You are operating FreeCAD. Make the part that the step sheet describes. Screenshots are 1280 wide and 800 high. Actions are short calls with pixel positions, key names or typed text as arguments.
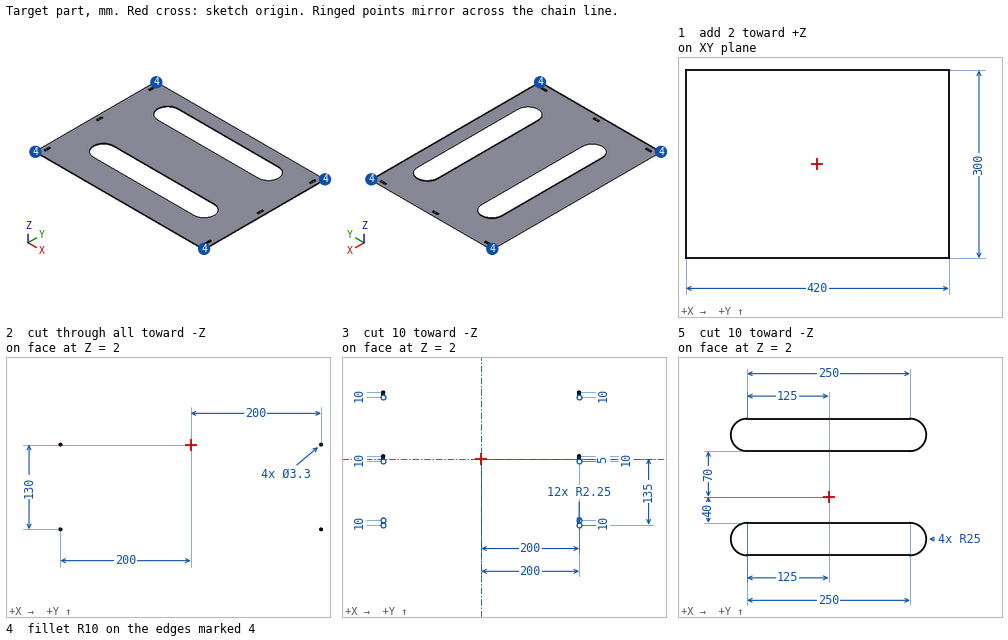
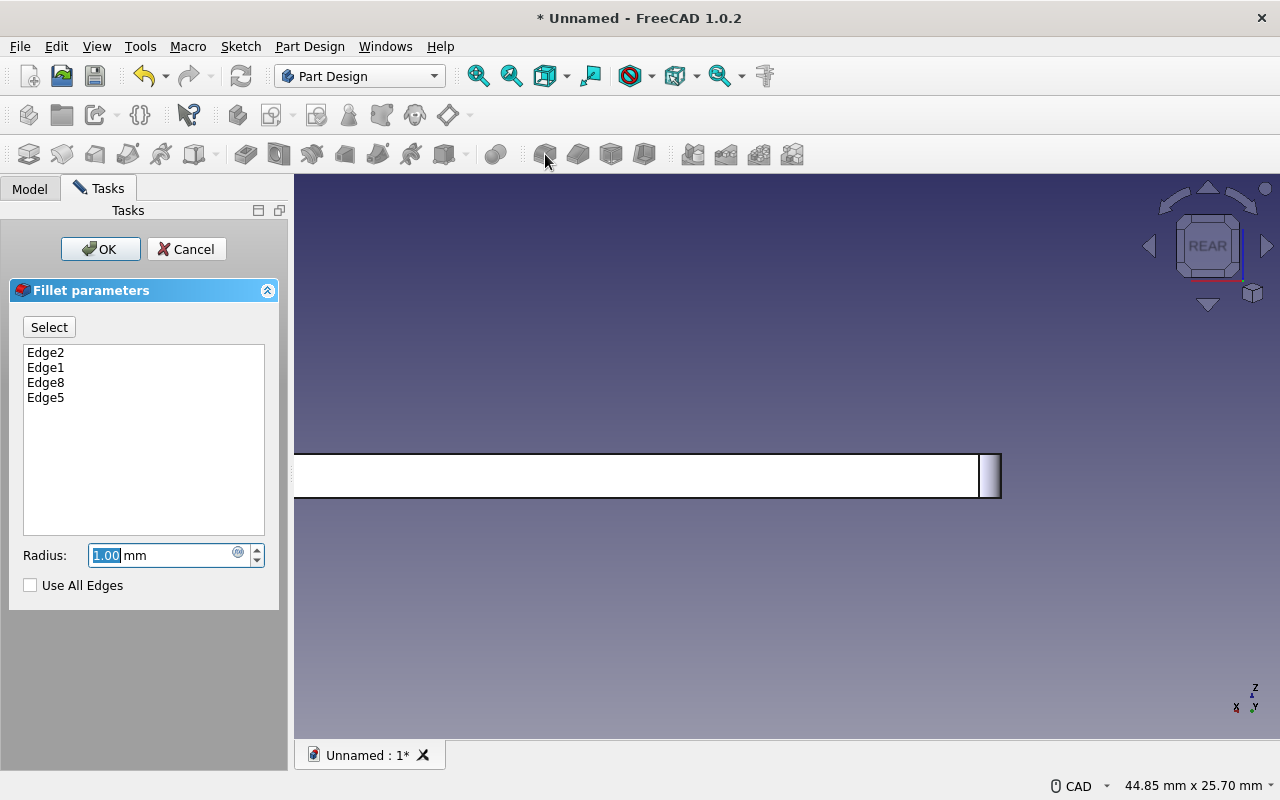
text(10)
key(Tab)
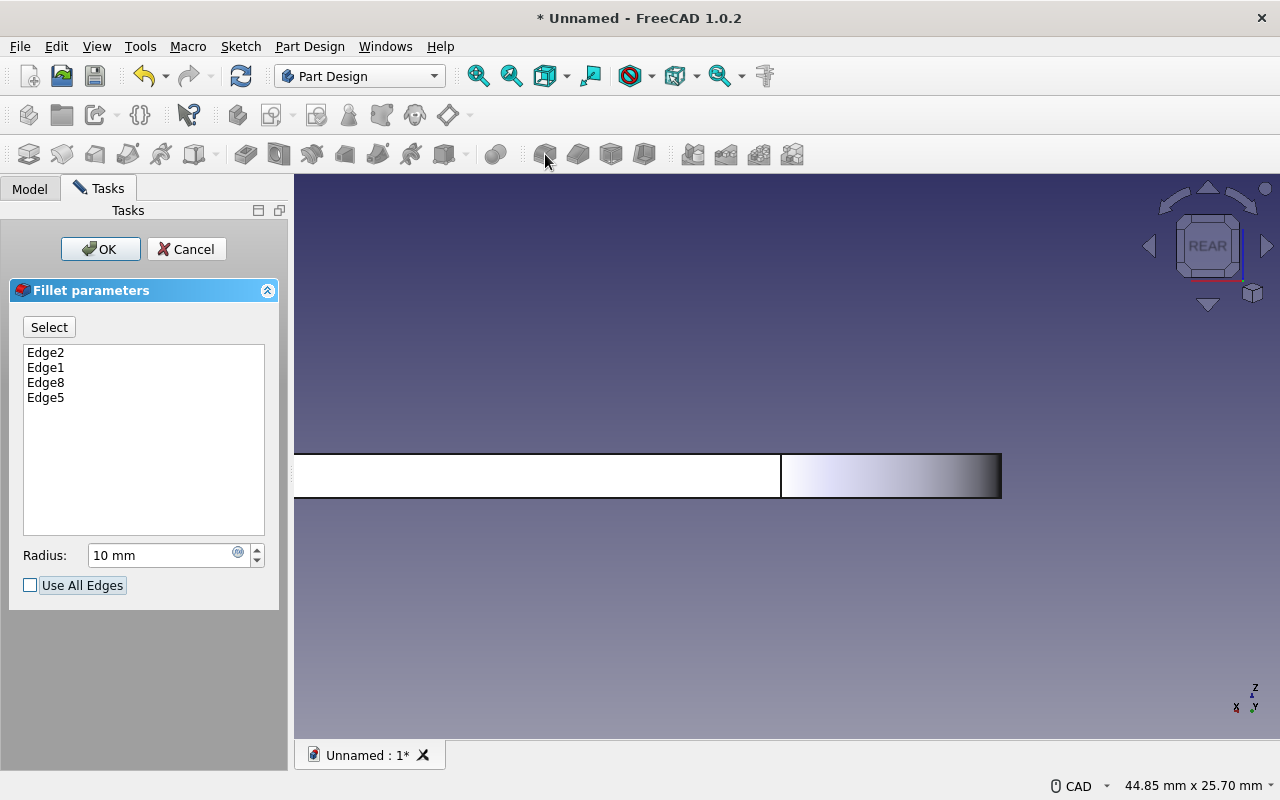
click(101, 249)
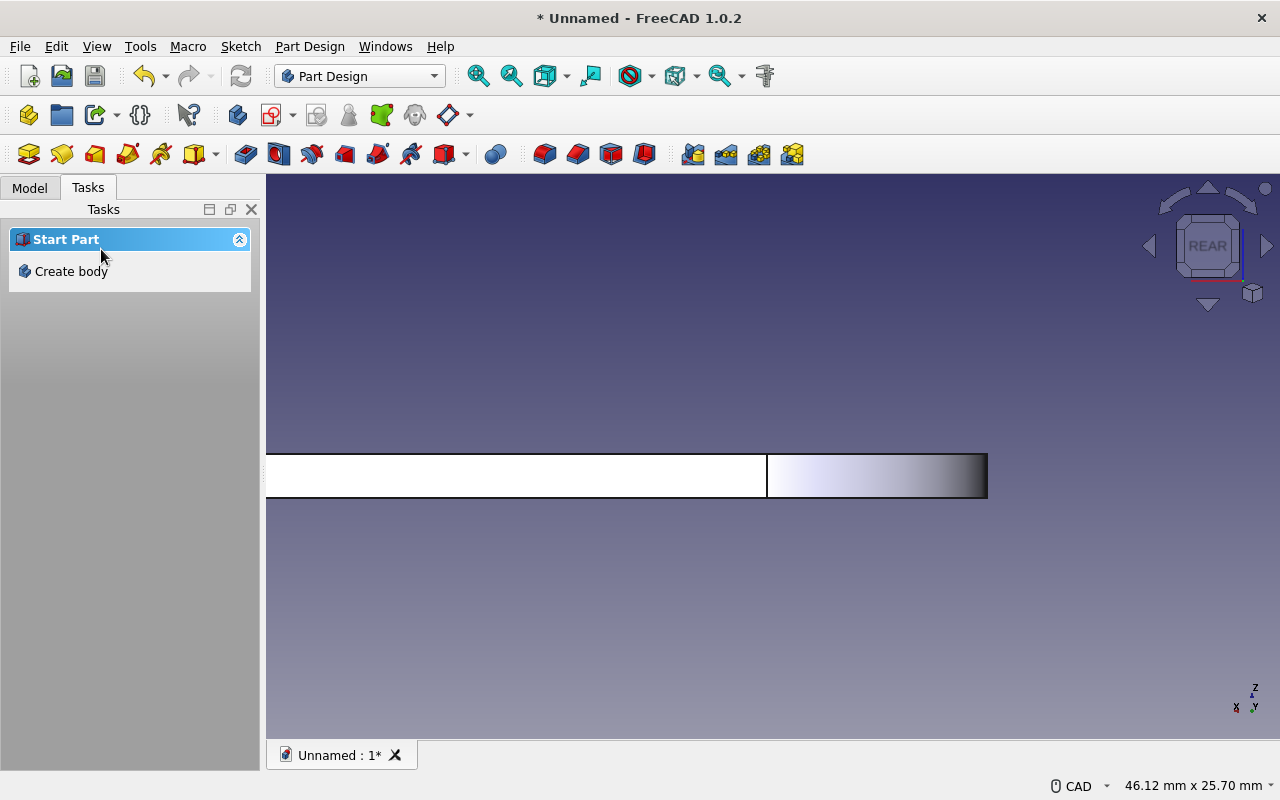
click(479, 76)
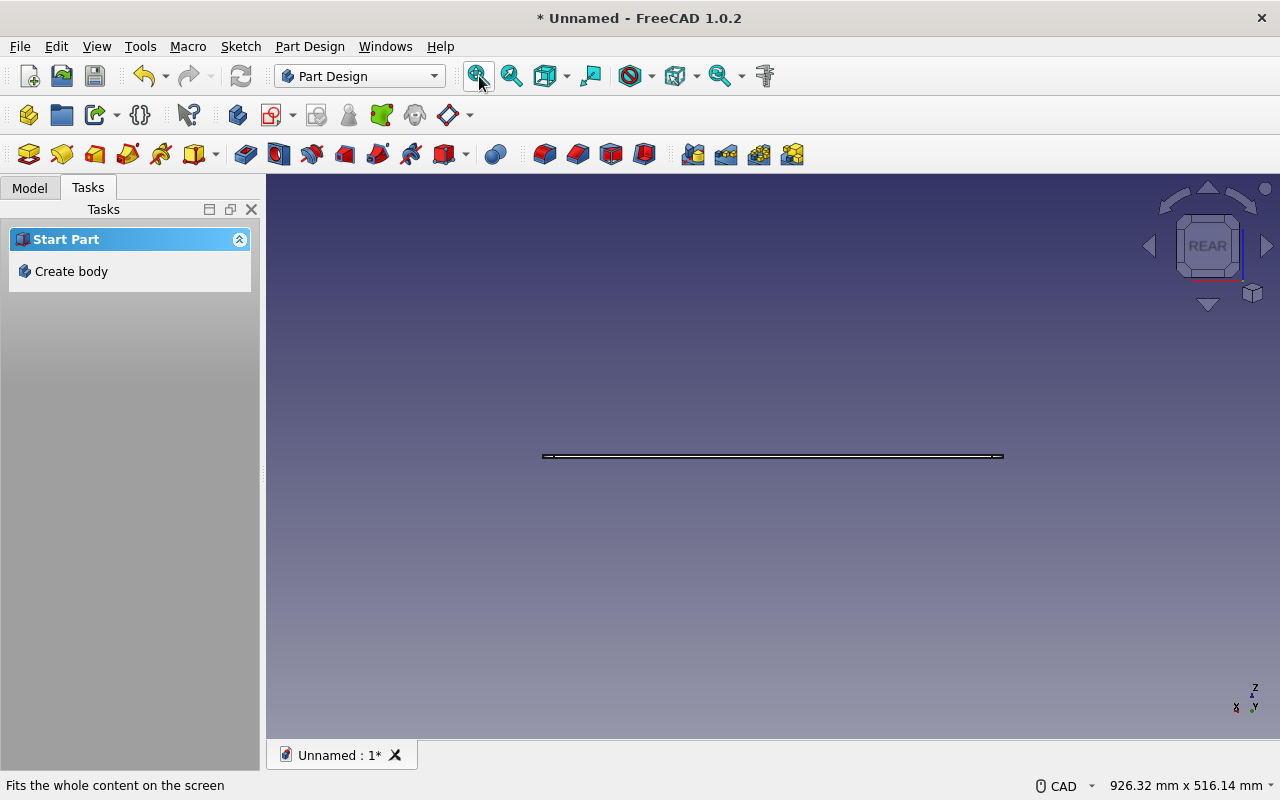
key(0)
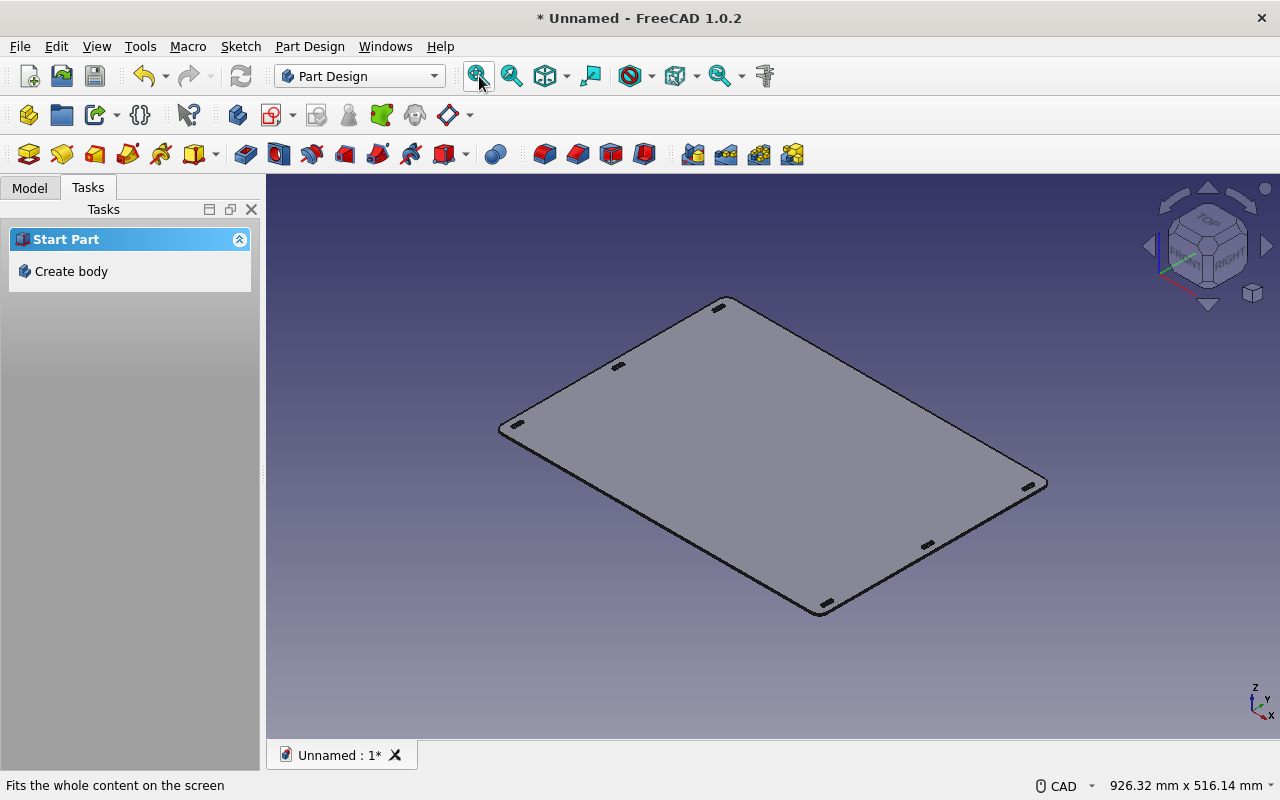
click(773, 455)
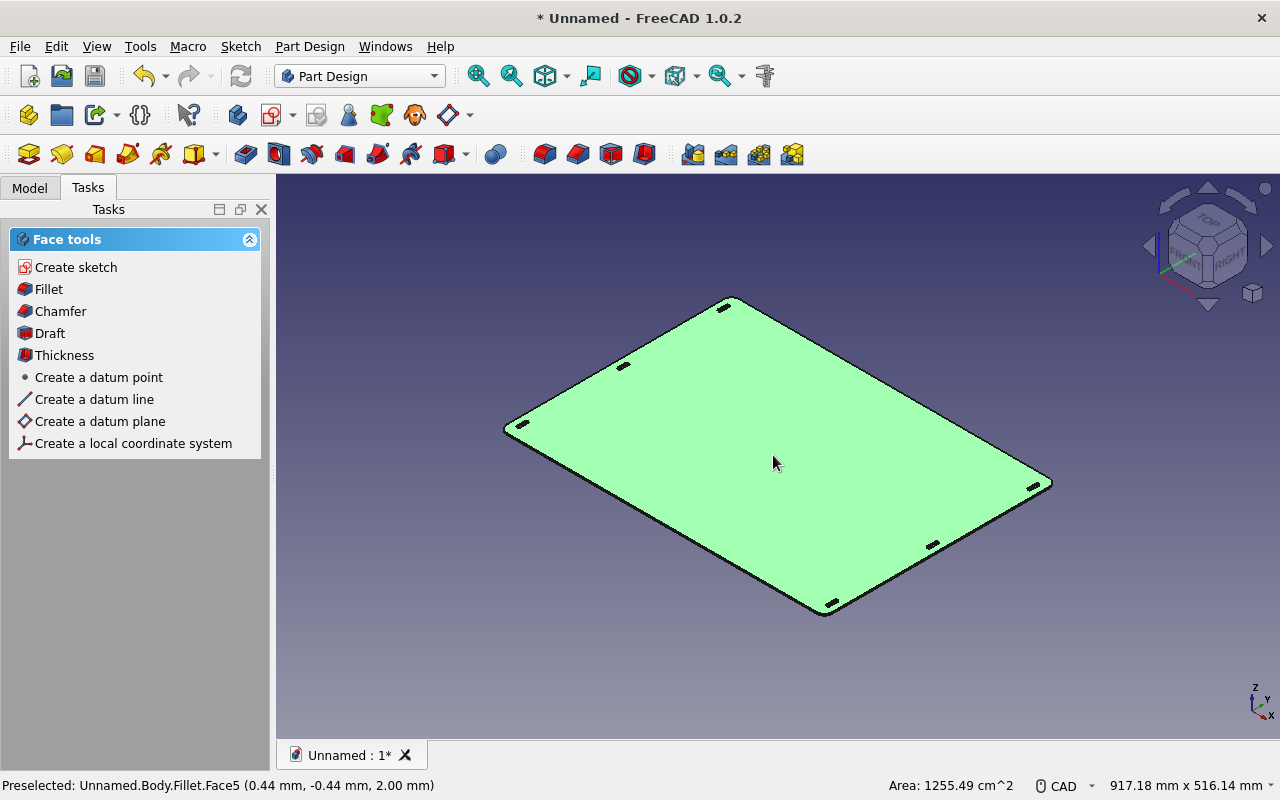
click(270, 116)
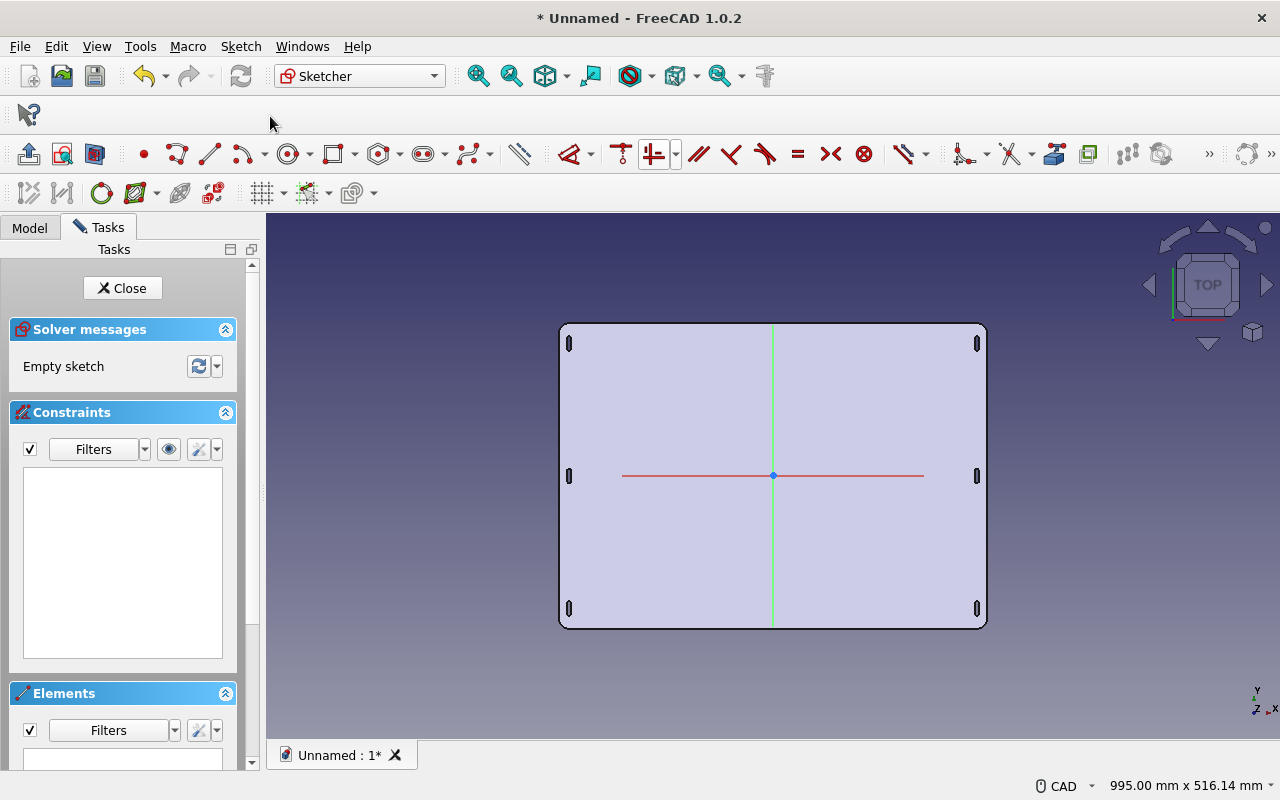
scroll(912, 430, up, 2)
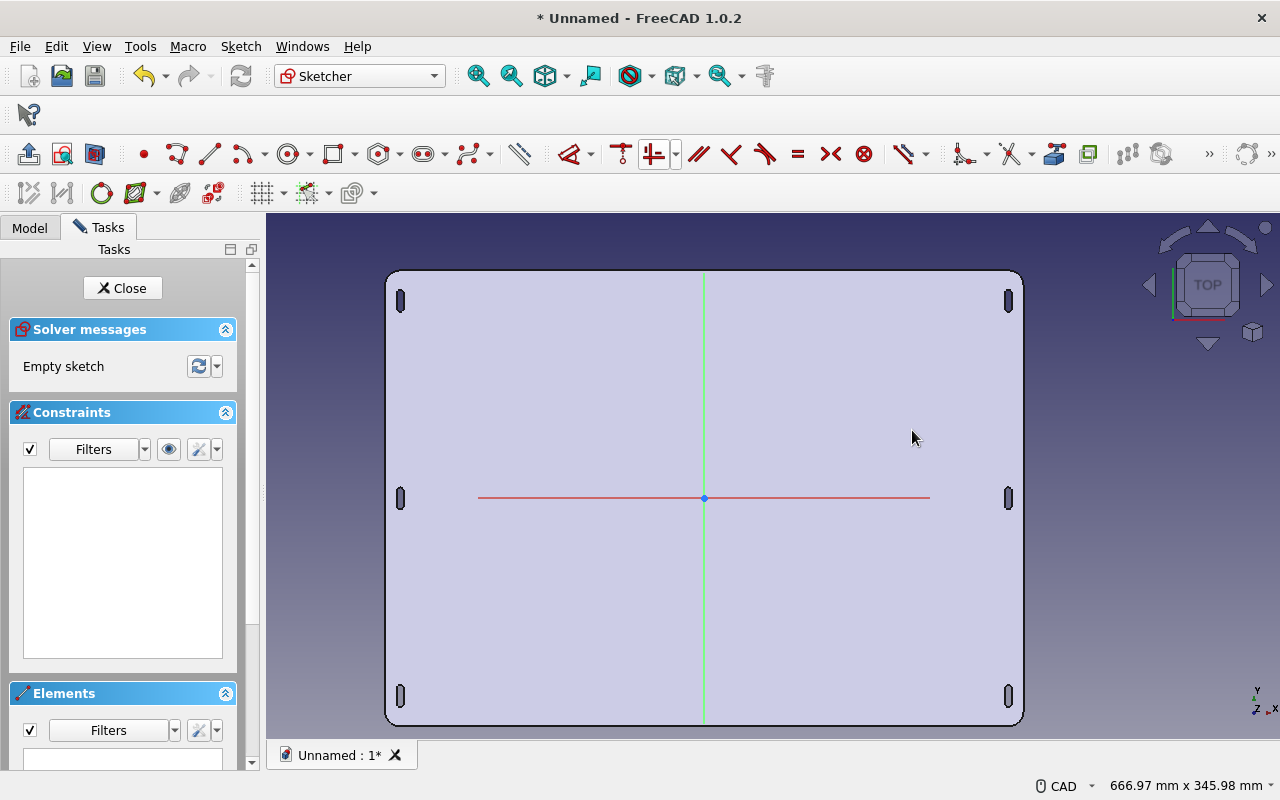
click(422, 154)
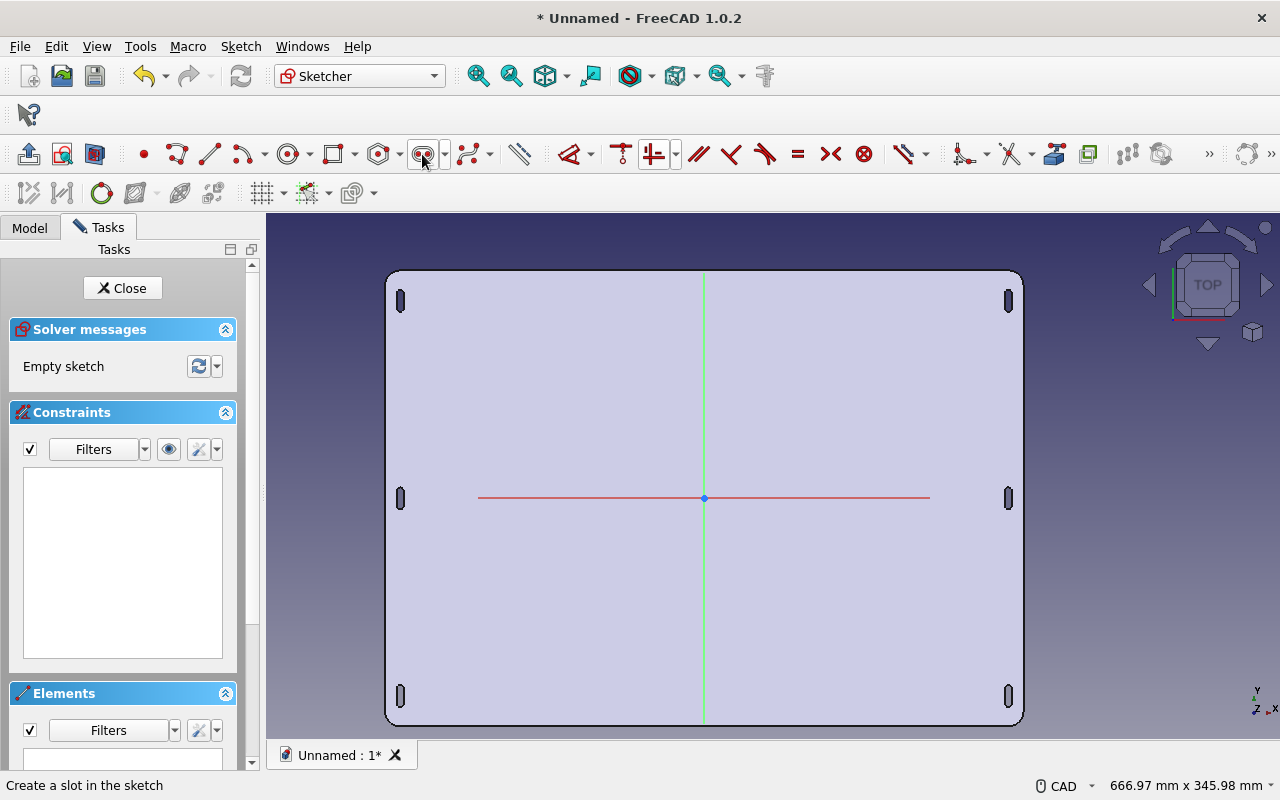
click(514, 597)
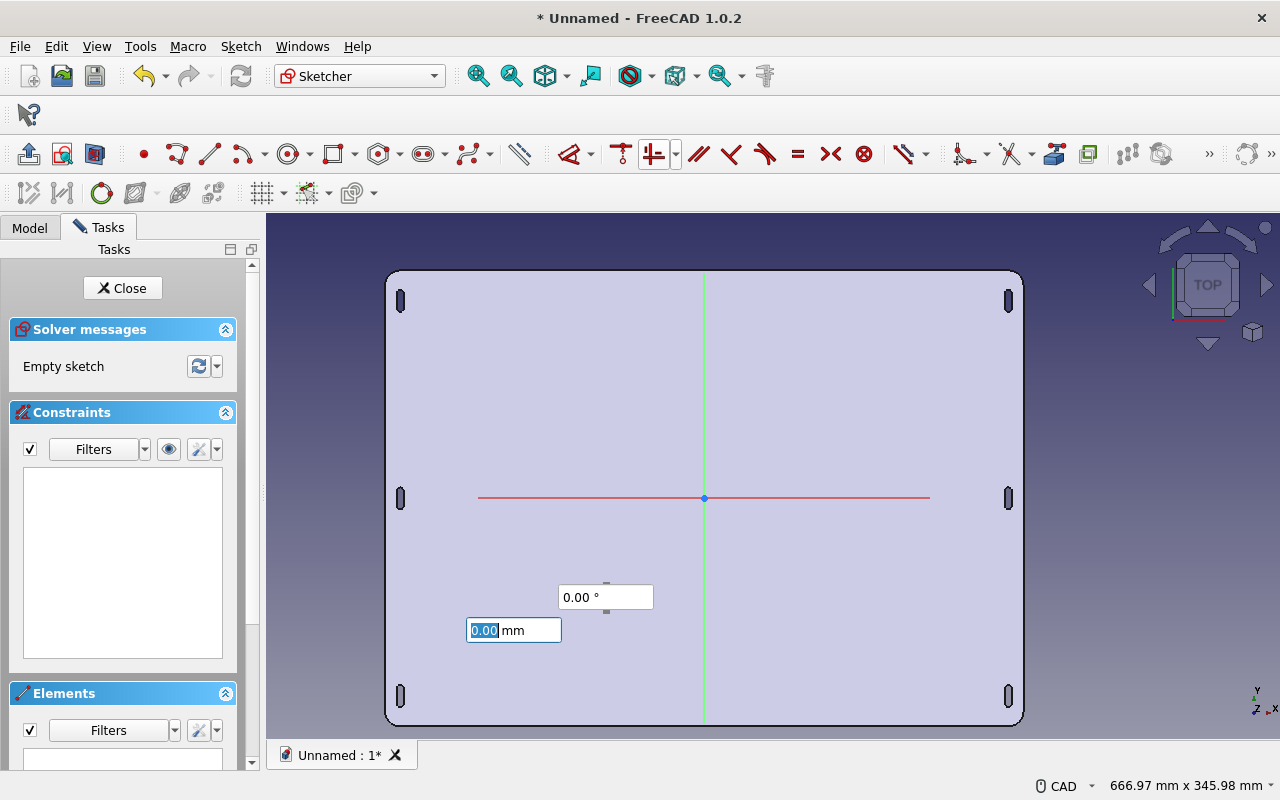
click(894, 597)